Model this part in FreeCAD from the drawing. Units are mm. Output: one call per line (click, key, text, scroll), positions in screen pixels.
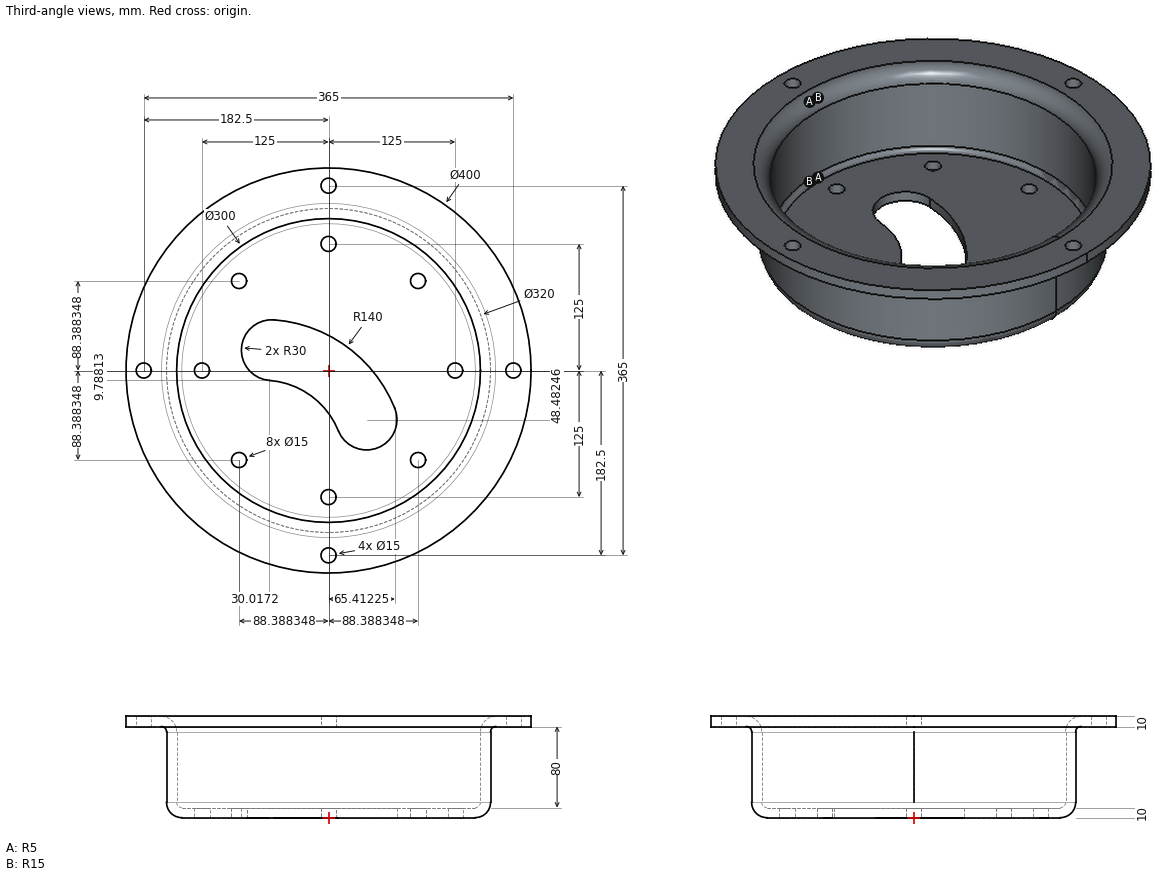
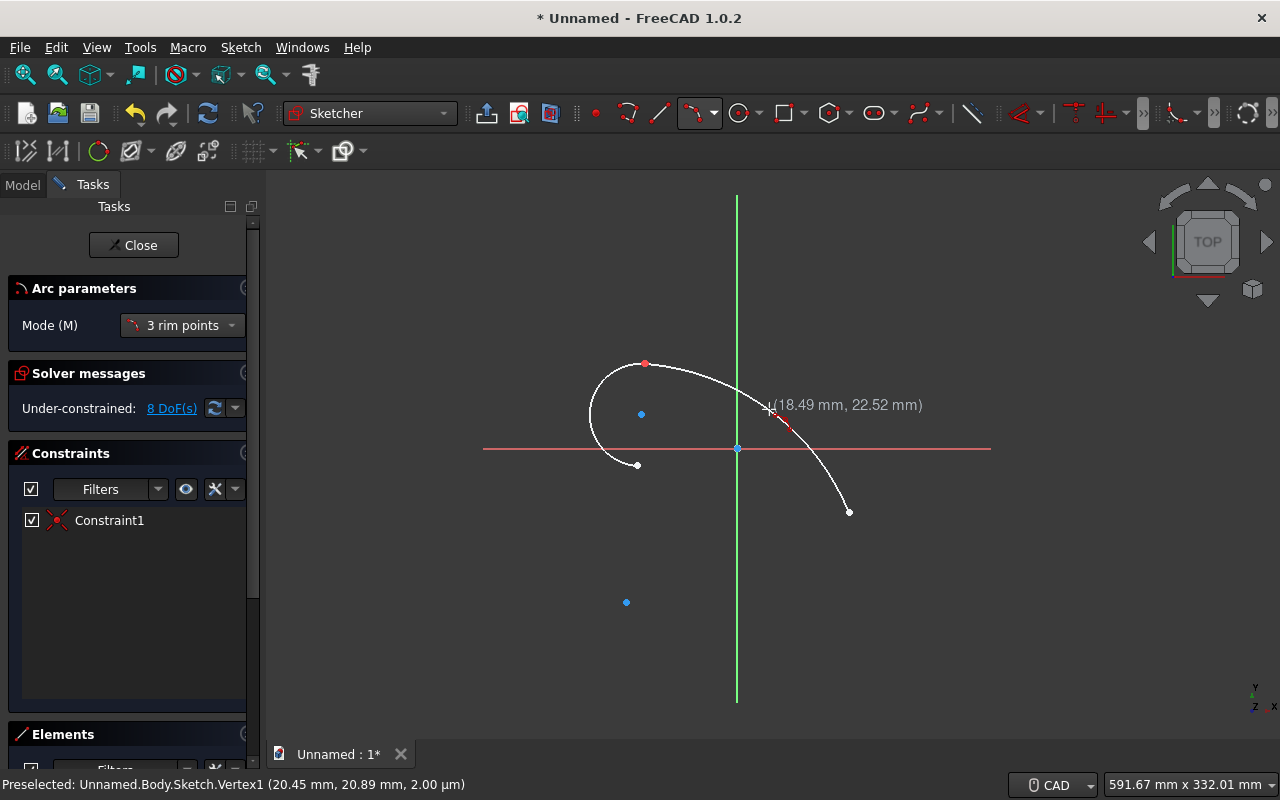
click(849, 513)
click(754, 551)
click(821, 579)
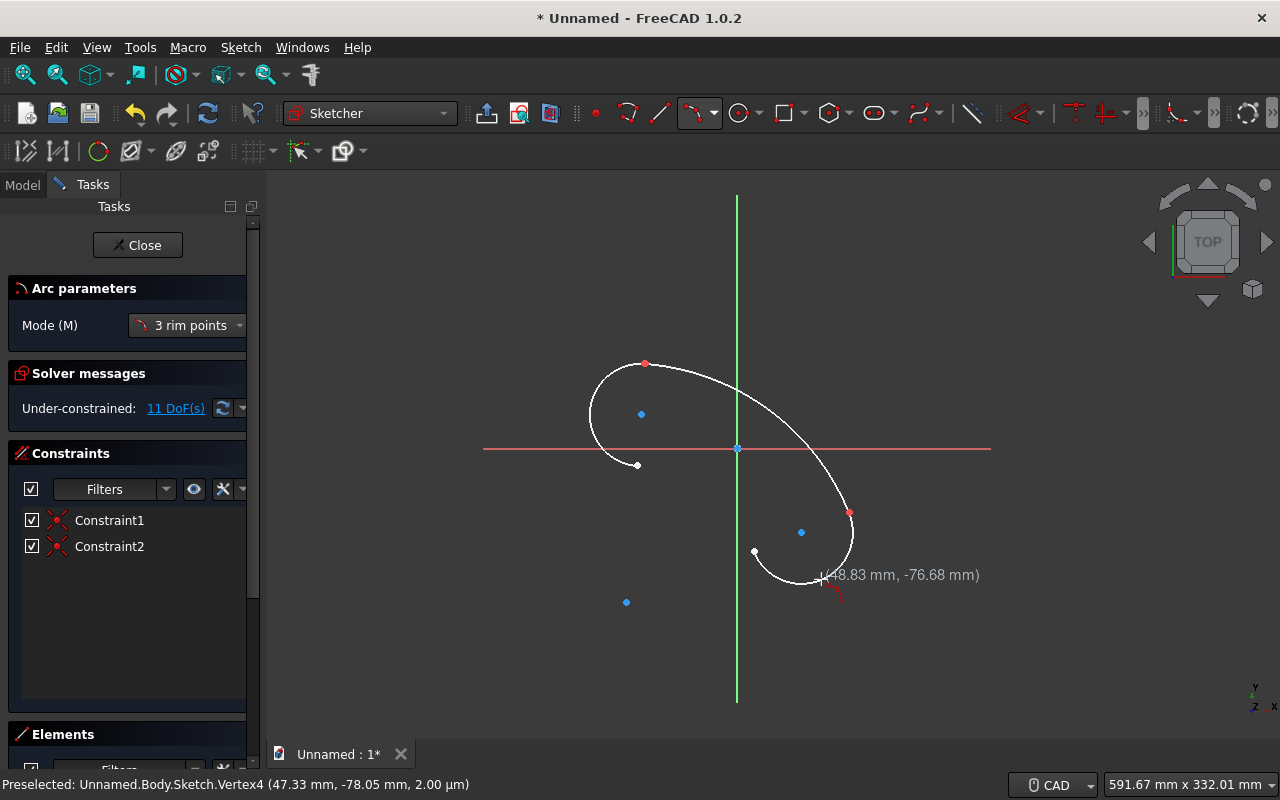
click(754, 552)
click(637, 466)
click(708, 491)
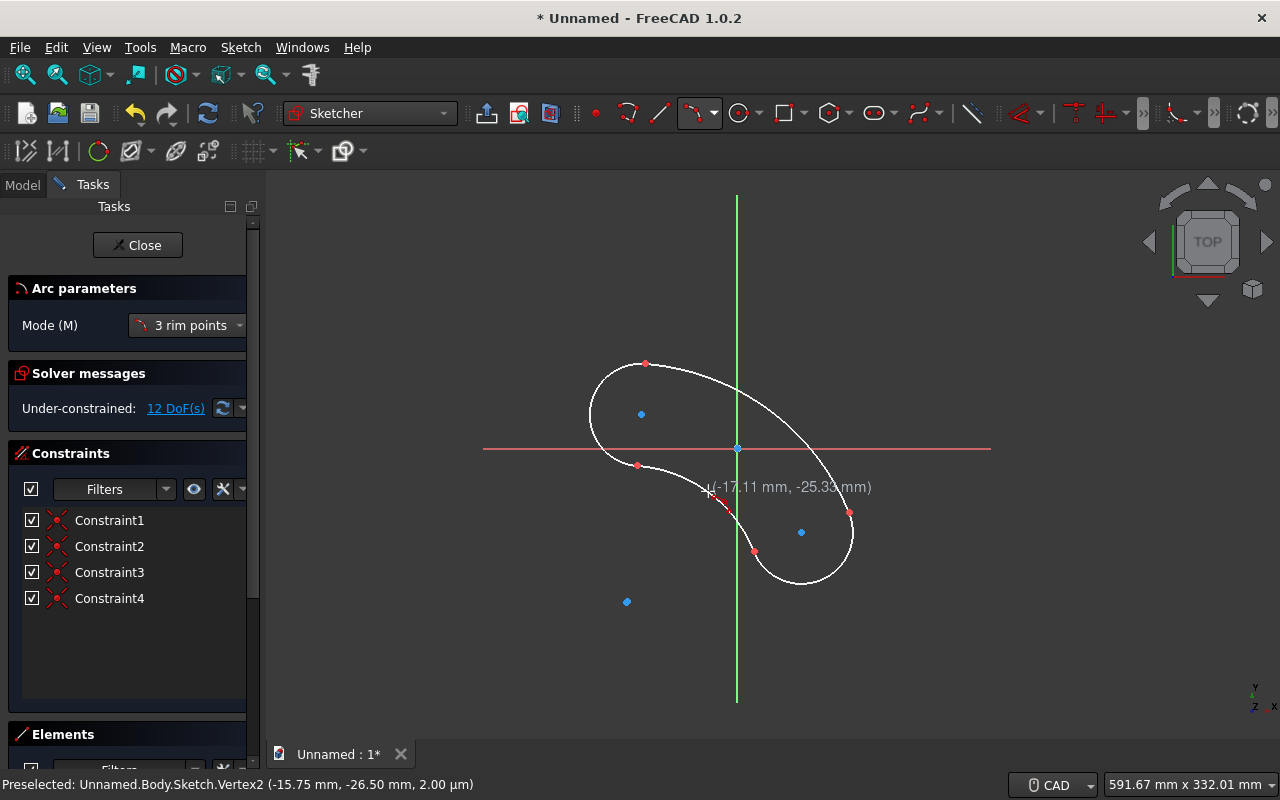
click(740, 114)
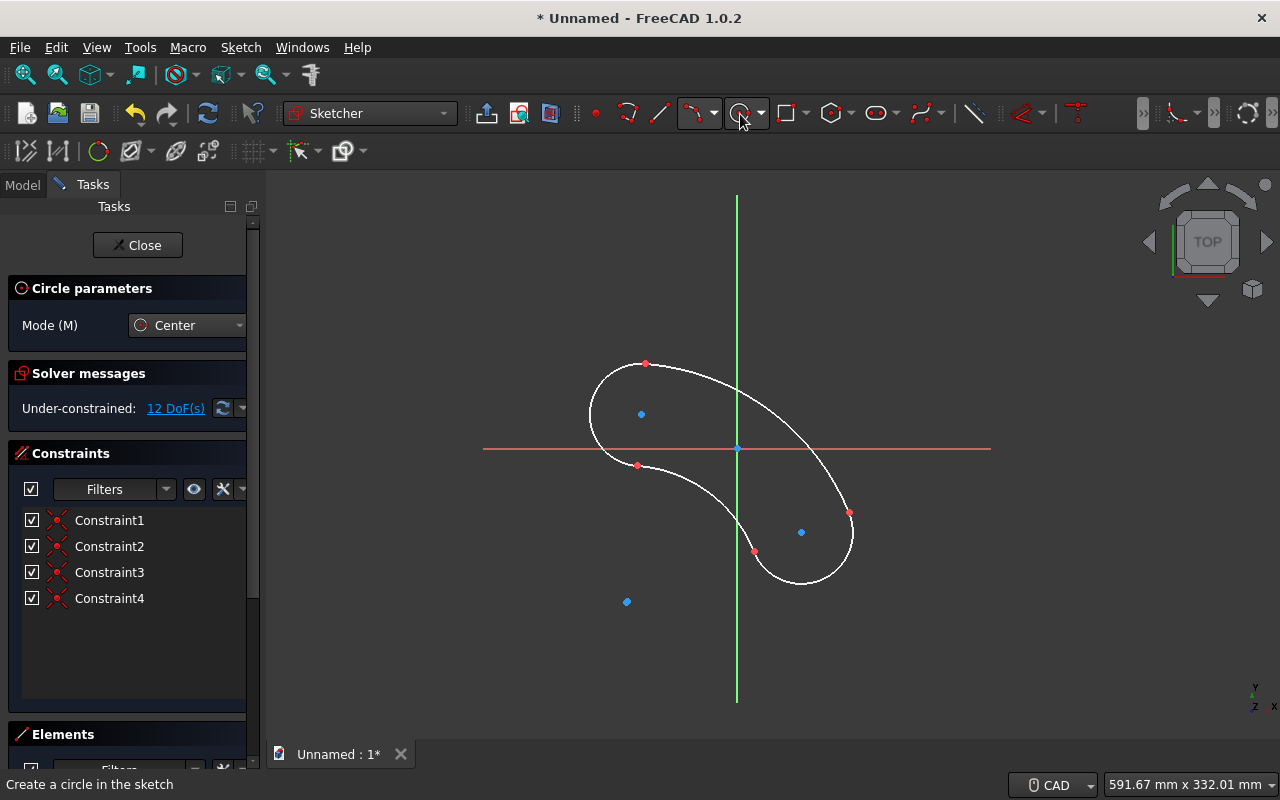
click(737, 449)
click(931, 255)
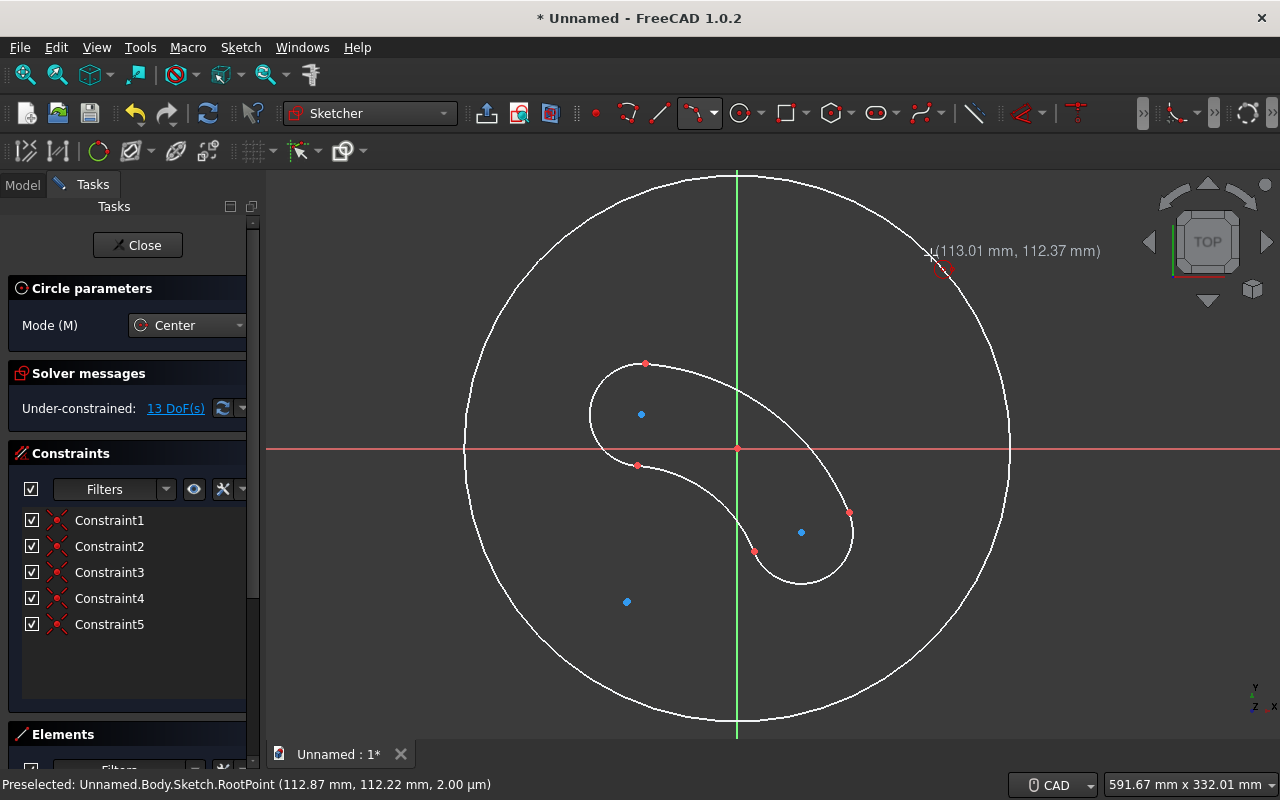
scroll(586, 600, up, 3)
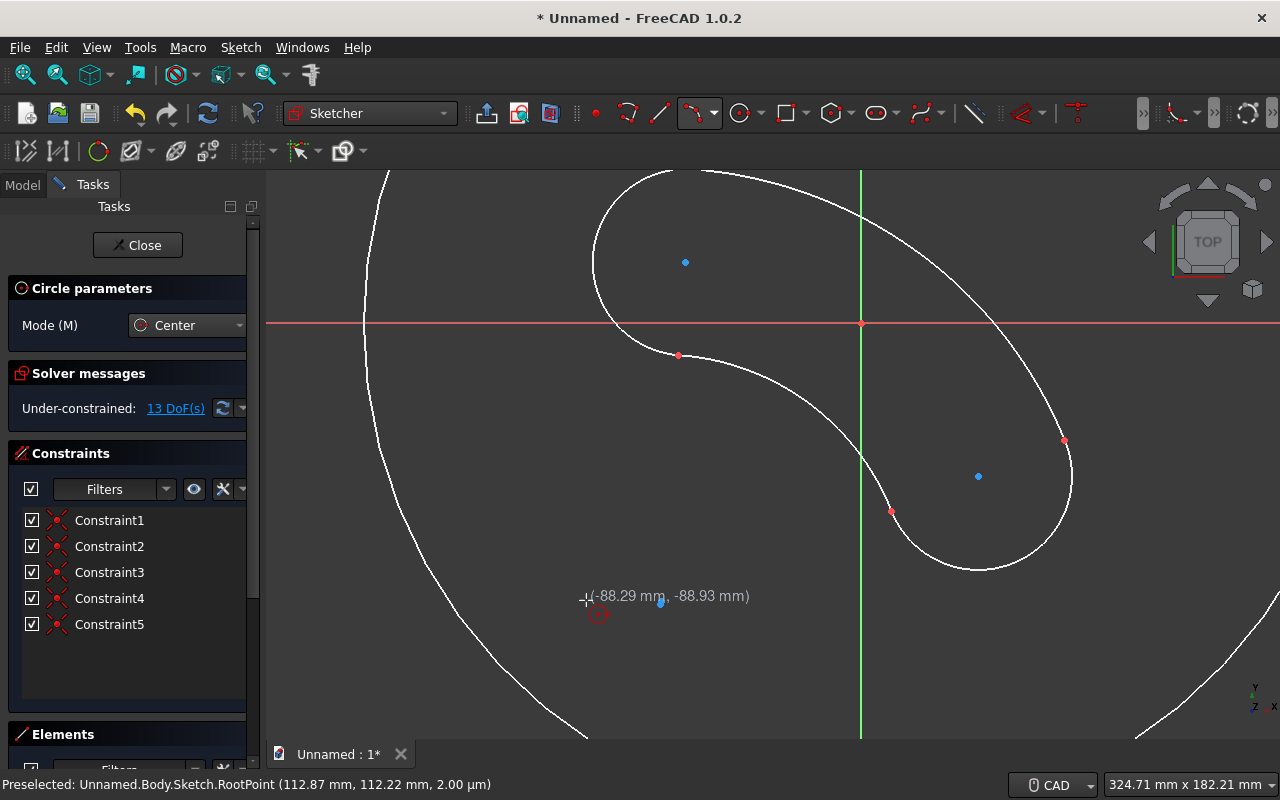
click(585, 600)
click(602, 583)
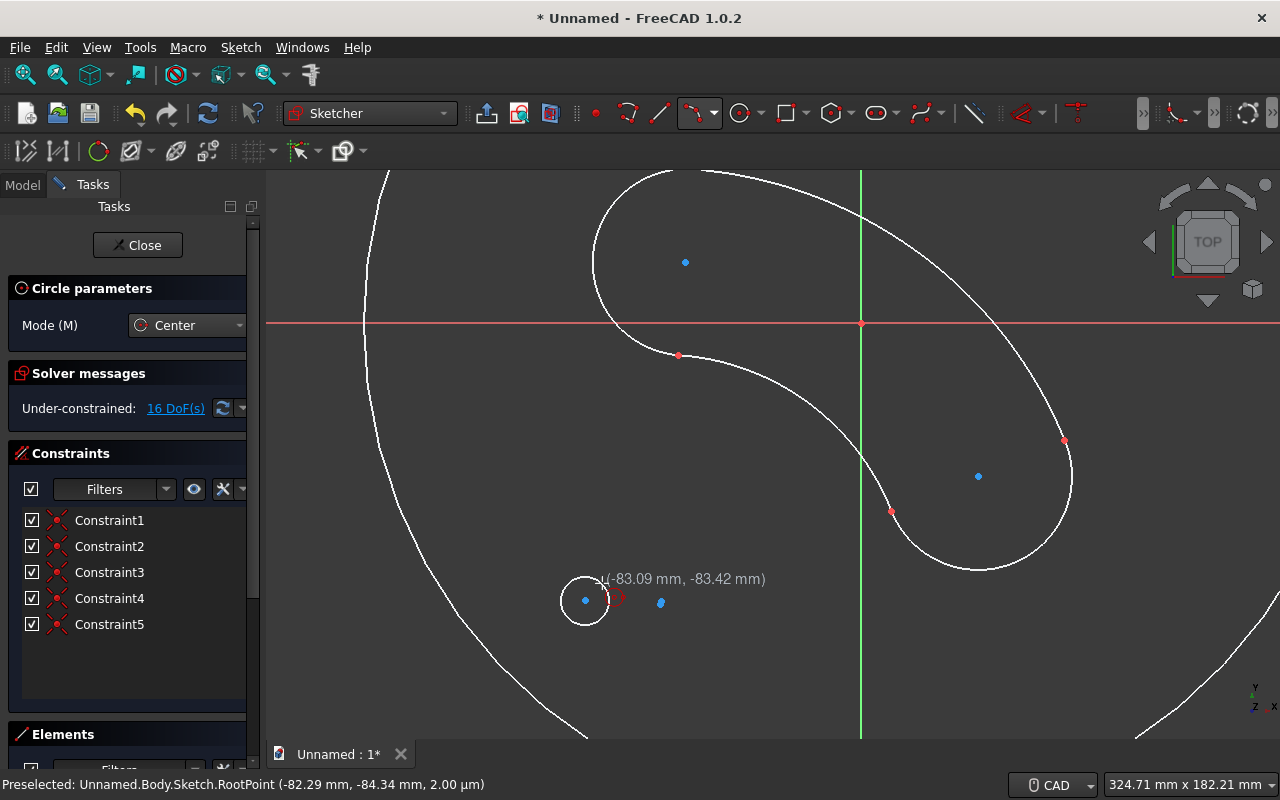
scroll(613, 531, down, 5)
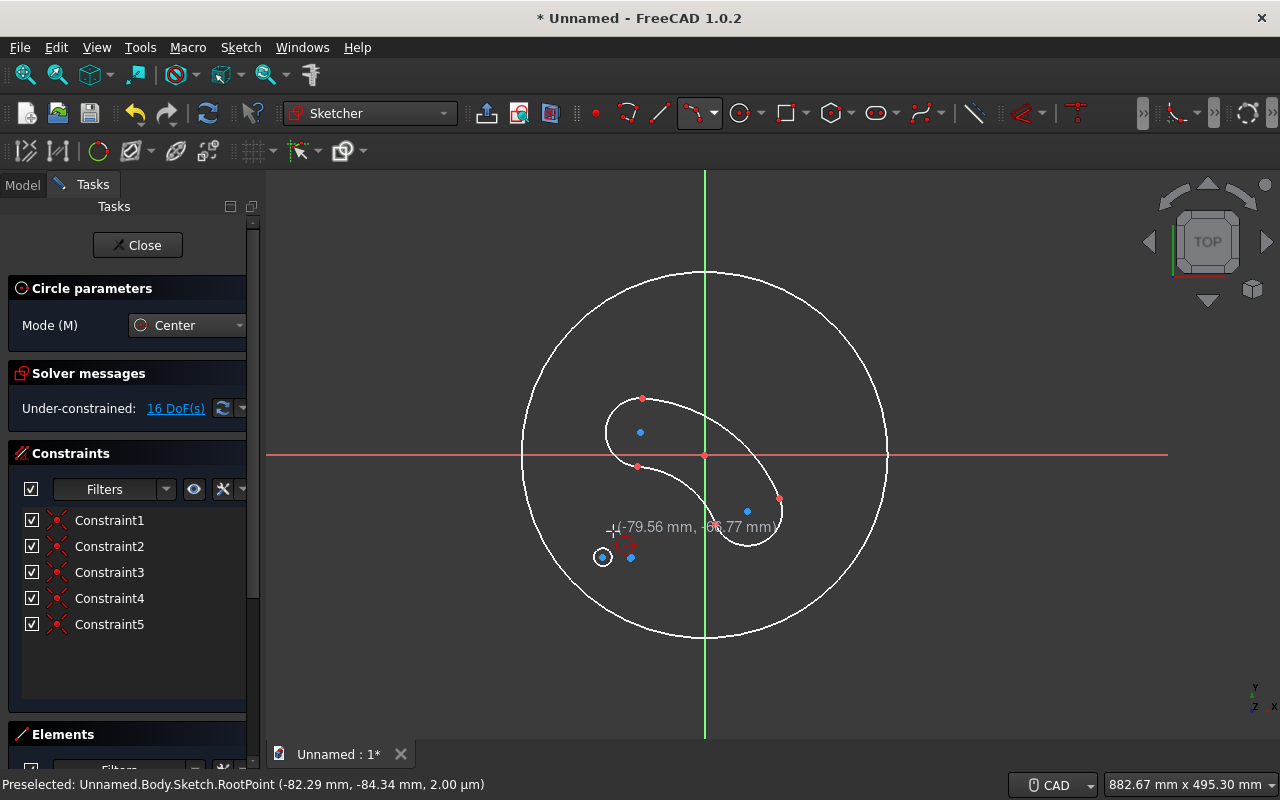
scroll(705, 599, up, 5)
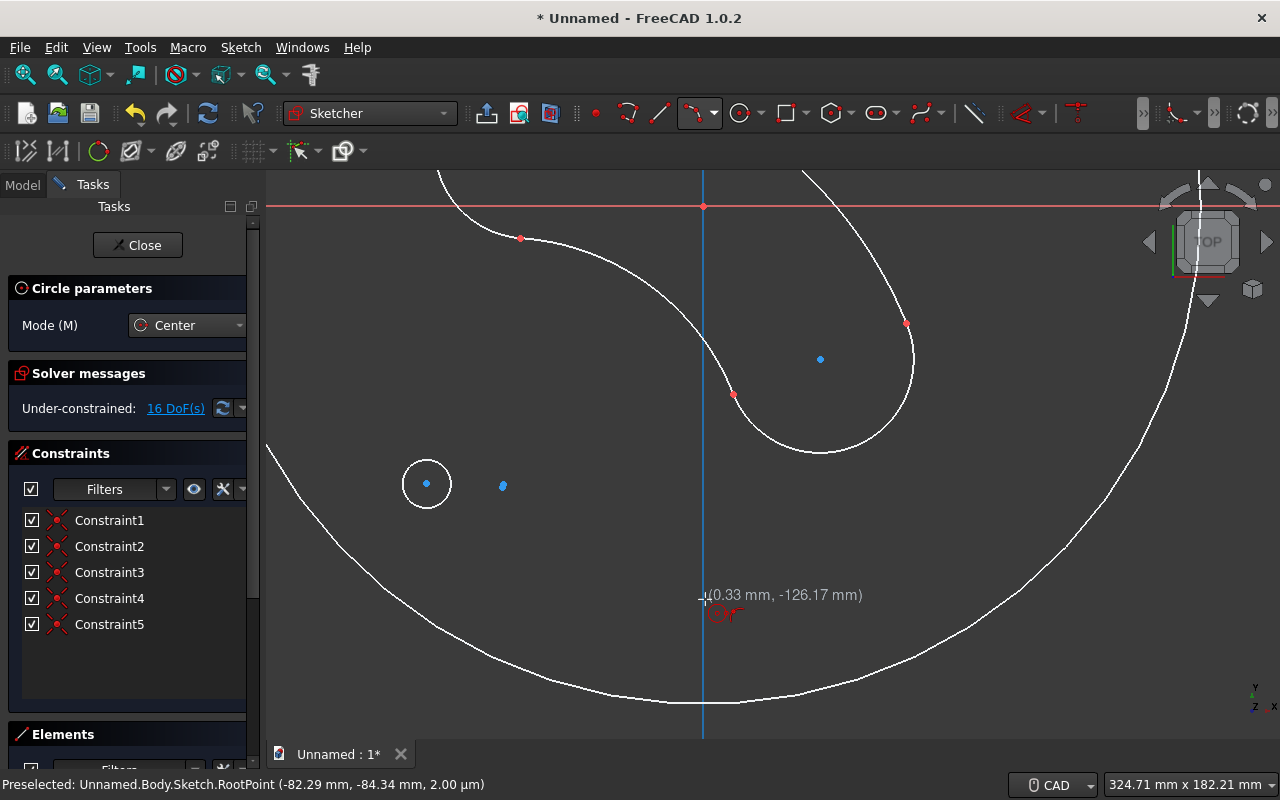
click(703, 597)
click(720, 580)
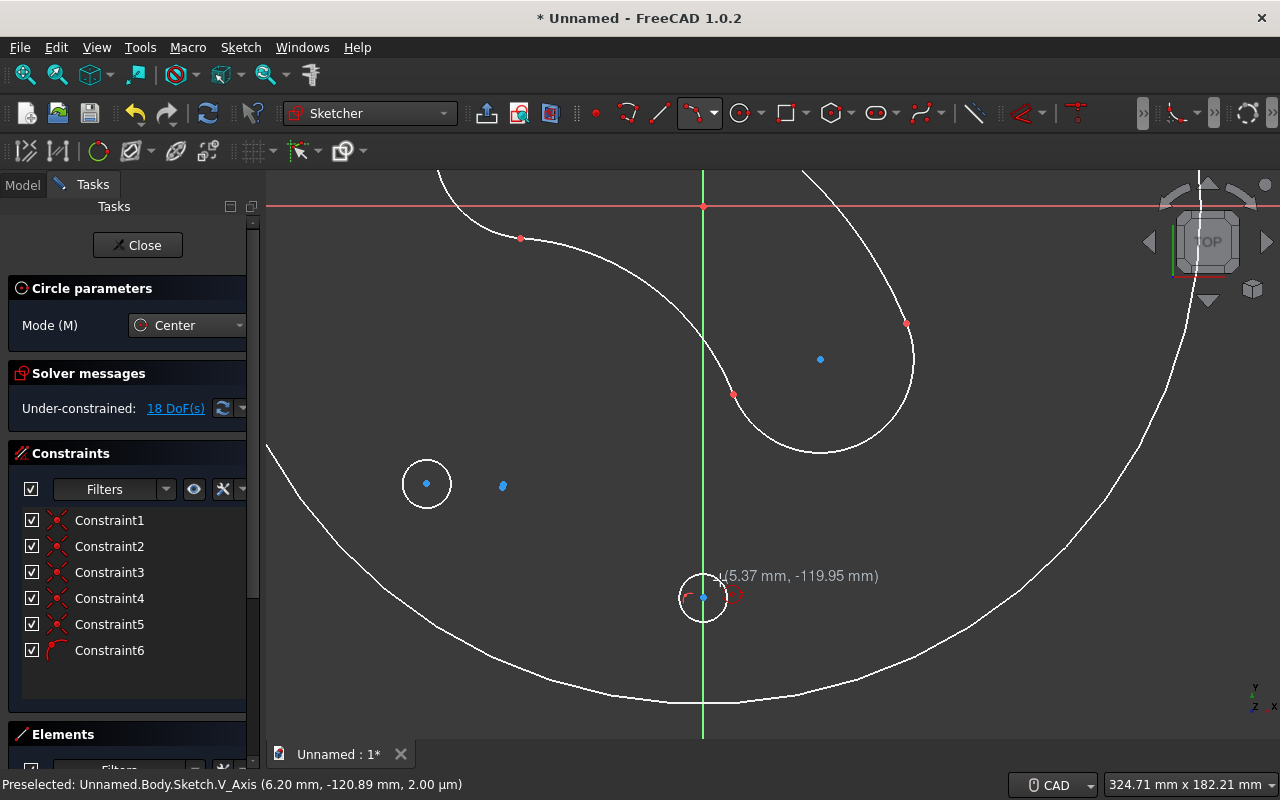
click(979, 482)
click(996, 466)